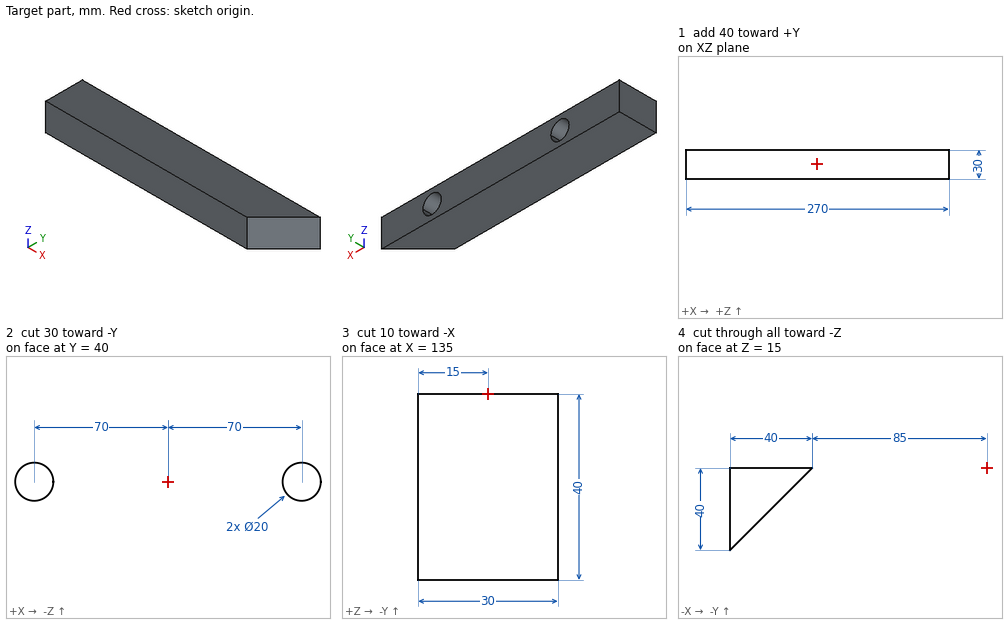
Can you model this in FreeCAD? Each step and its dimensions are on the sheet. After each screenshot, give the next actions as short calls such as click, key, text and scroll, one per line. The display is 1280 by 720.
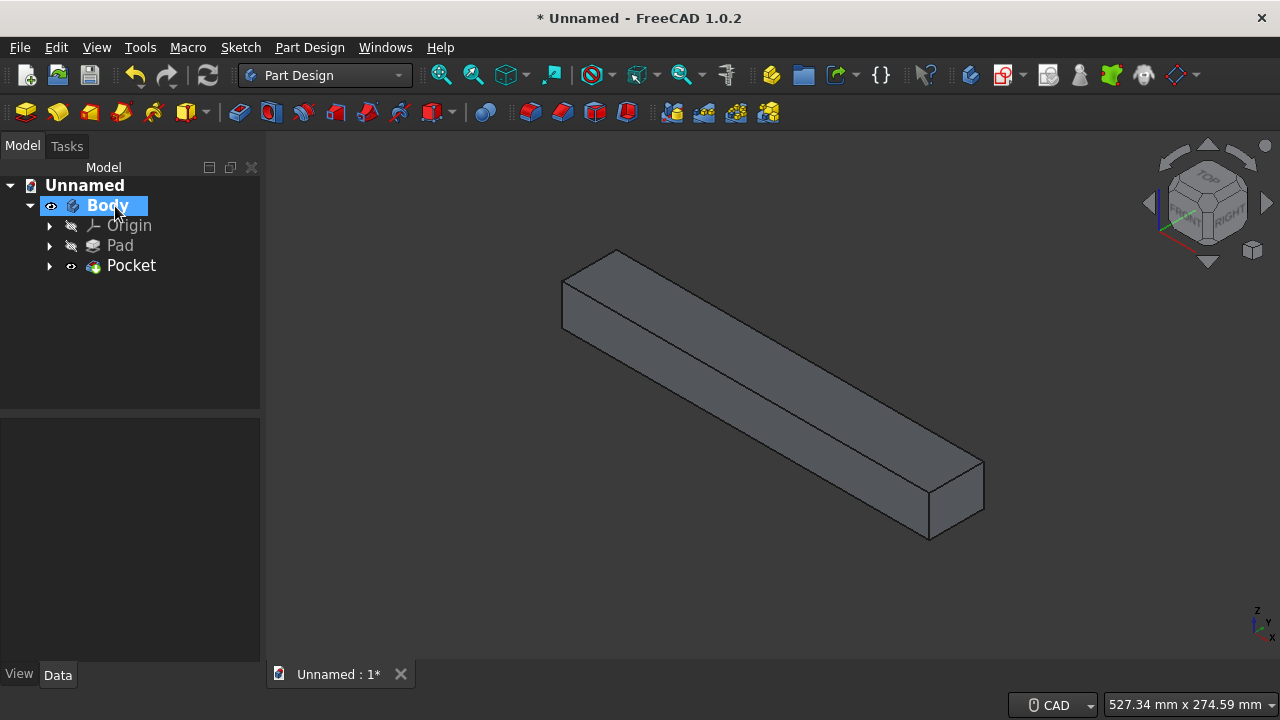
click(957, 500)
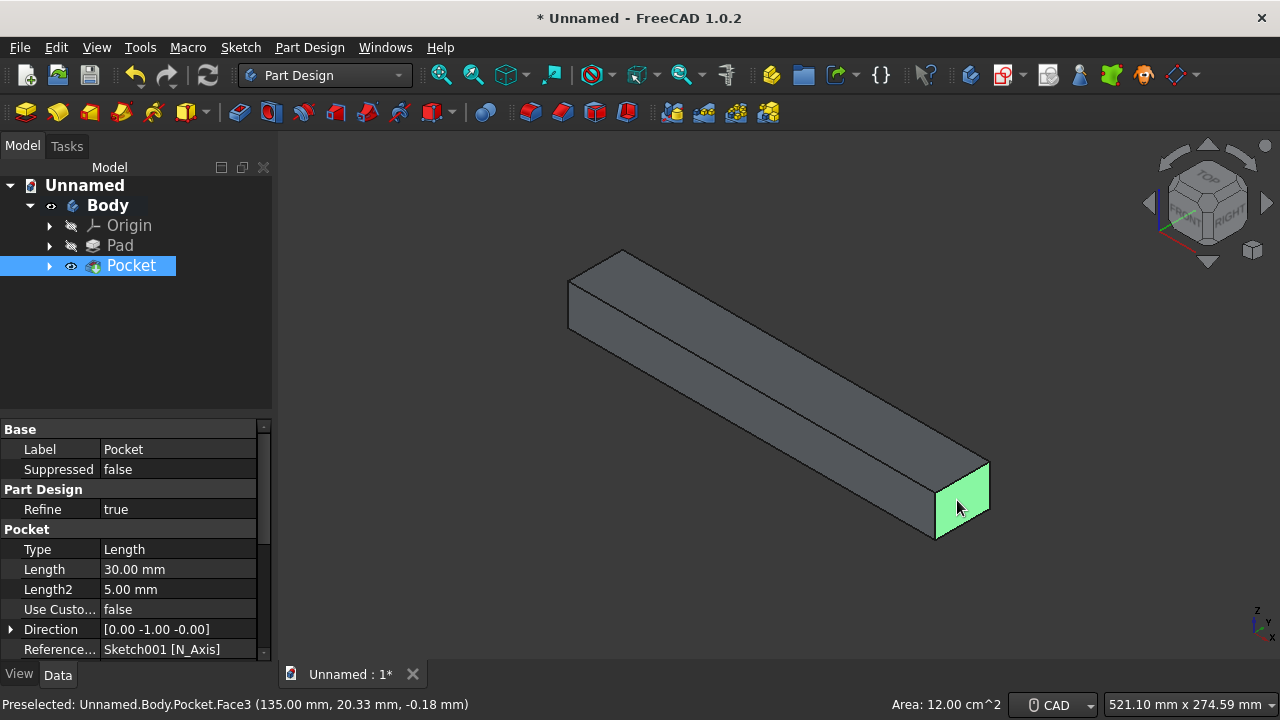
click(1004, 76)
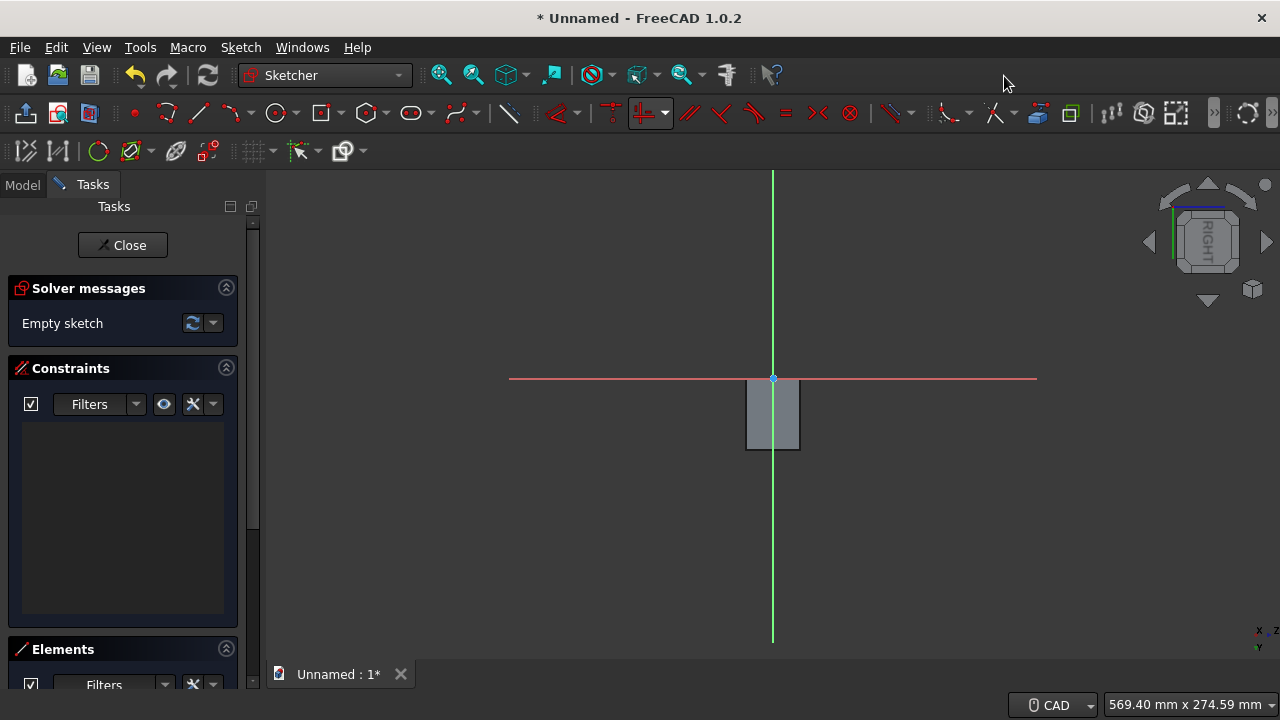
scroll(795, 415, up, 7)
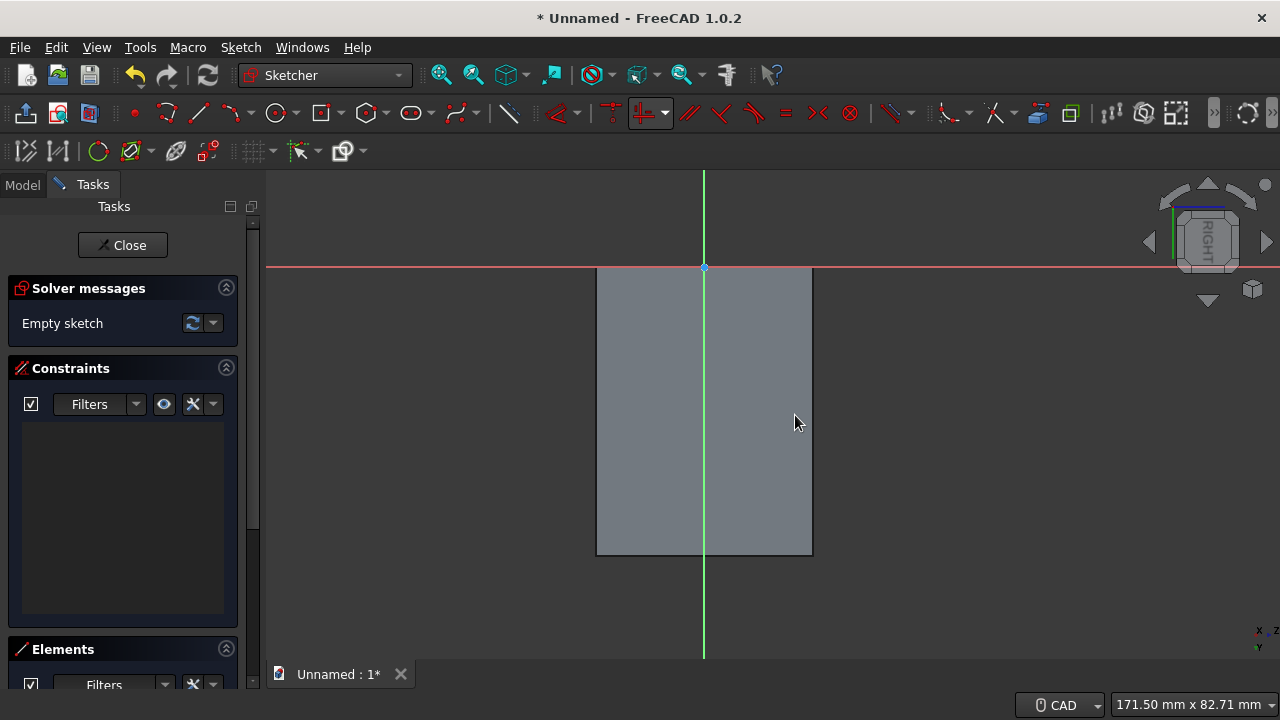
click(344, 114)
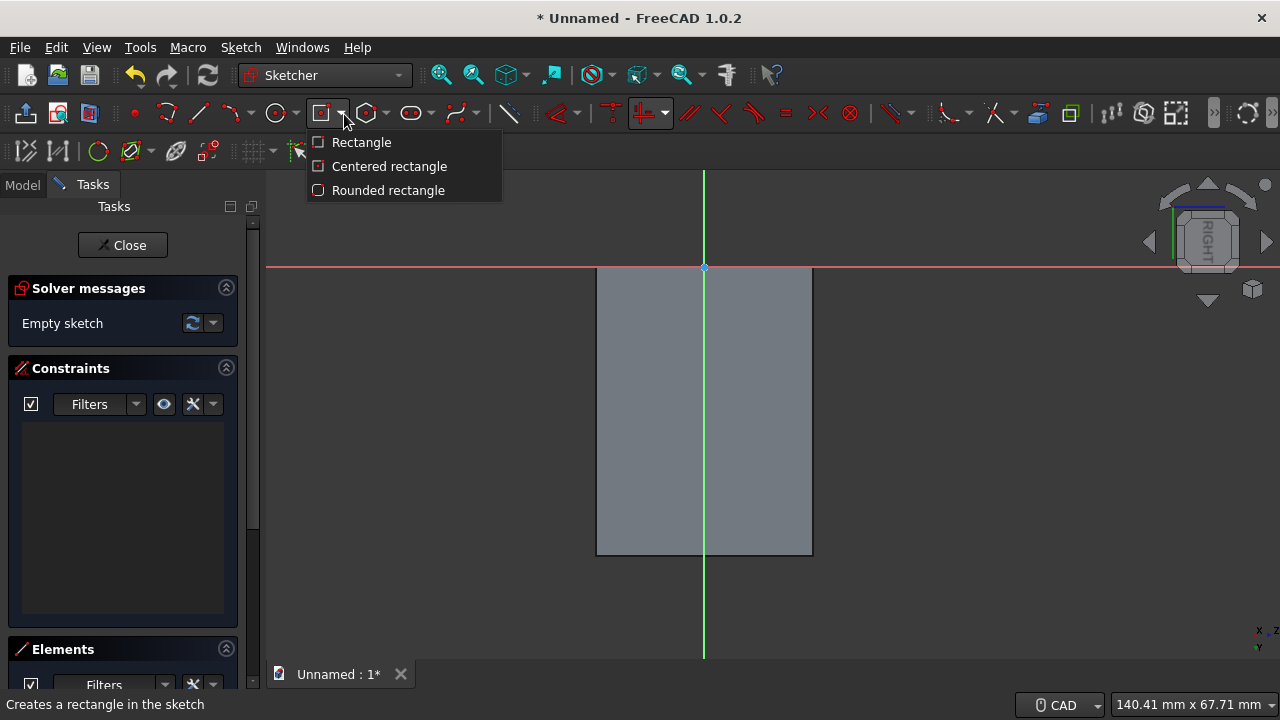
click(404, 142)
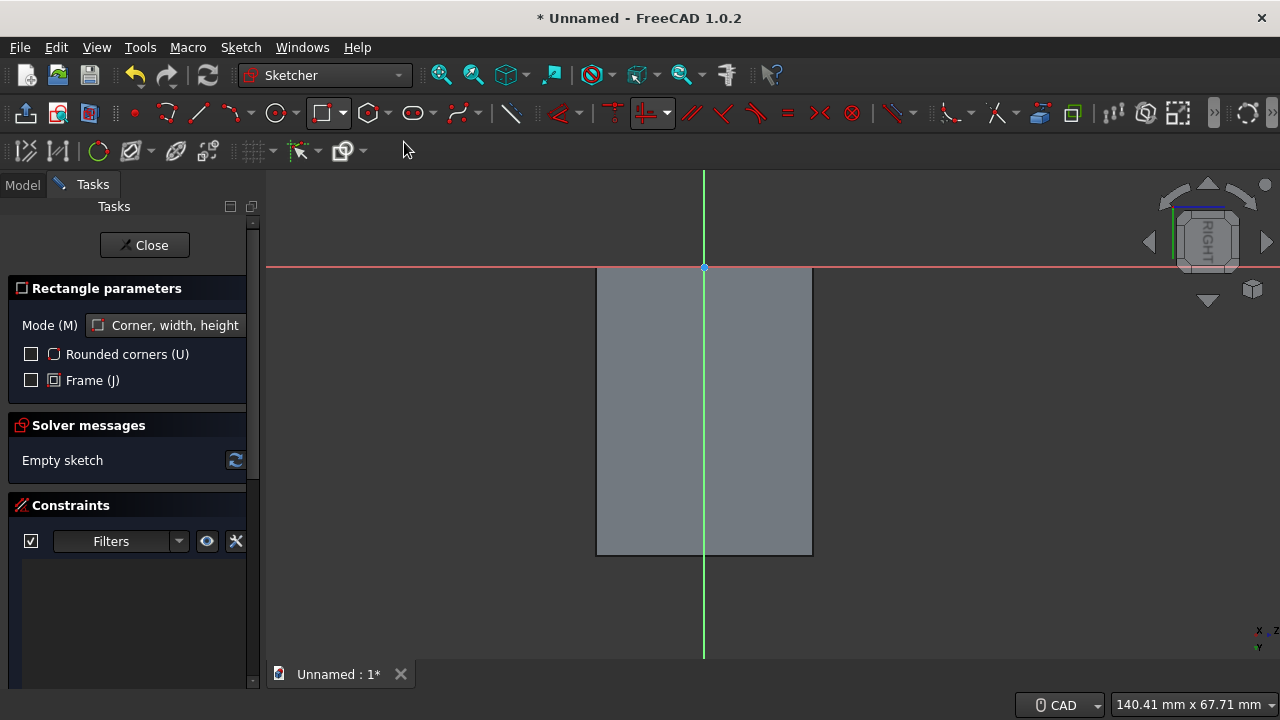
click(596, 267)
move(813, 556)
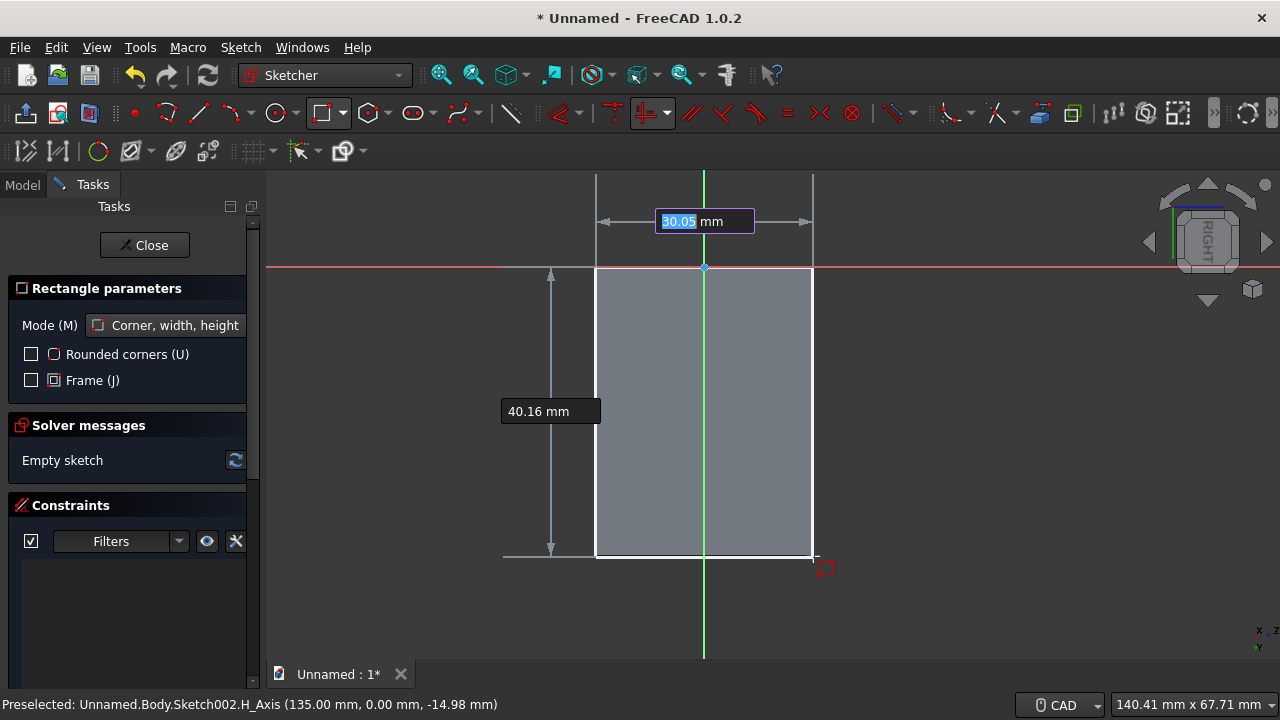
text(30)
key(Tab)
text(40)
key(Return)
key(Escape)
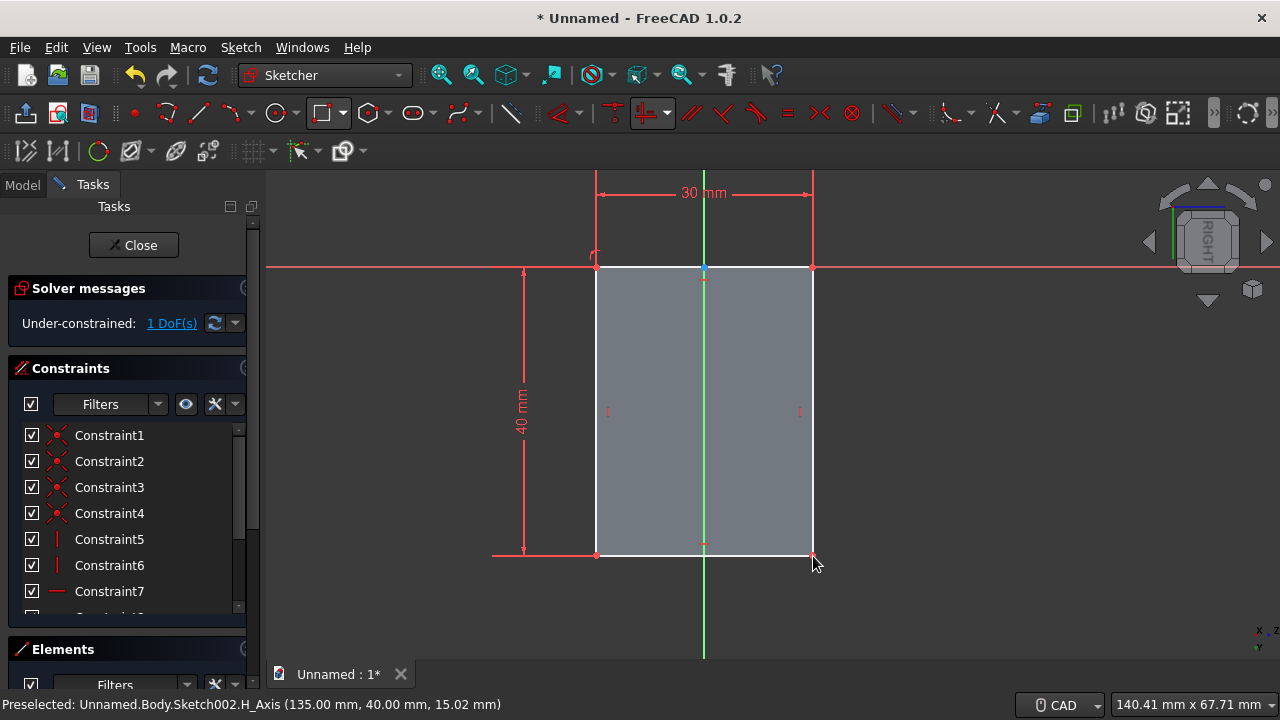
click(558, 114)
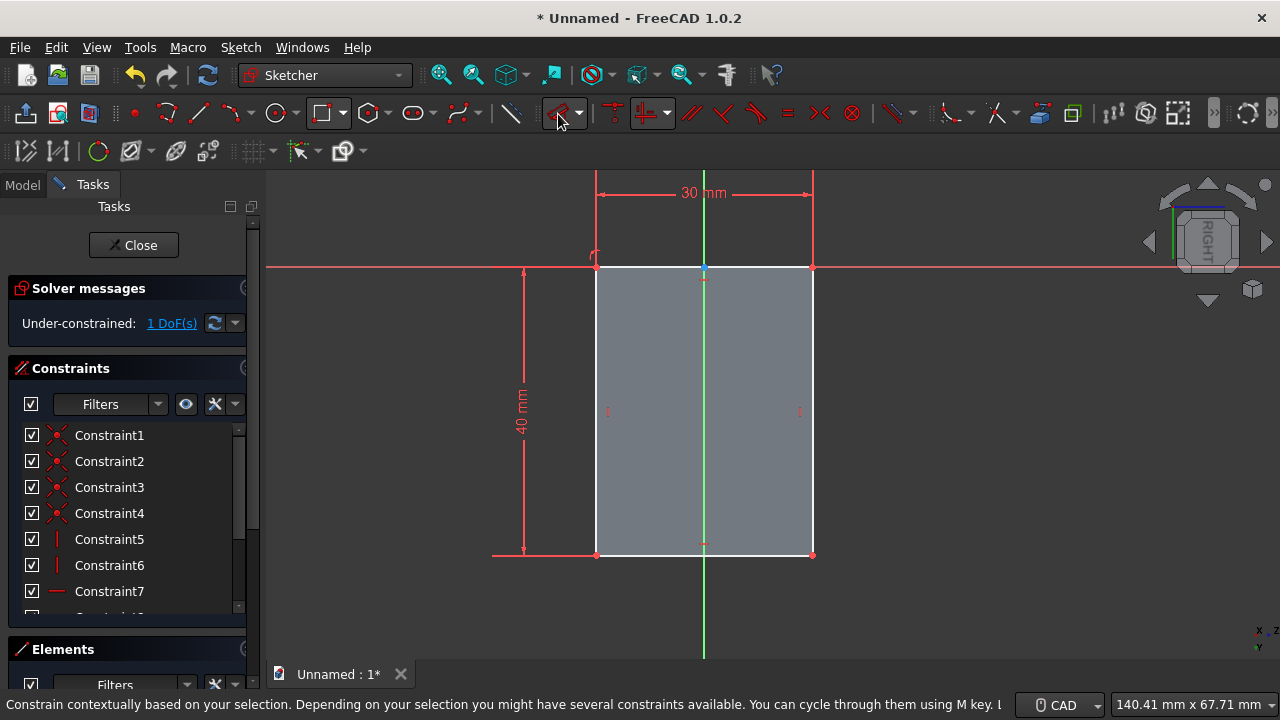
click(596, 267)
click(650, 233)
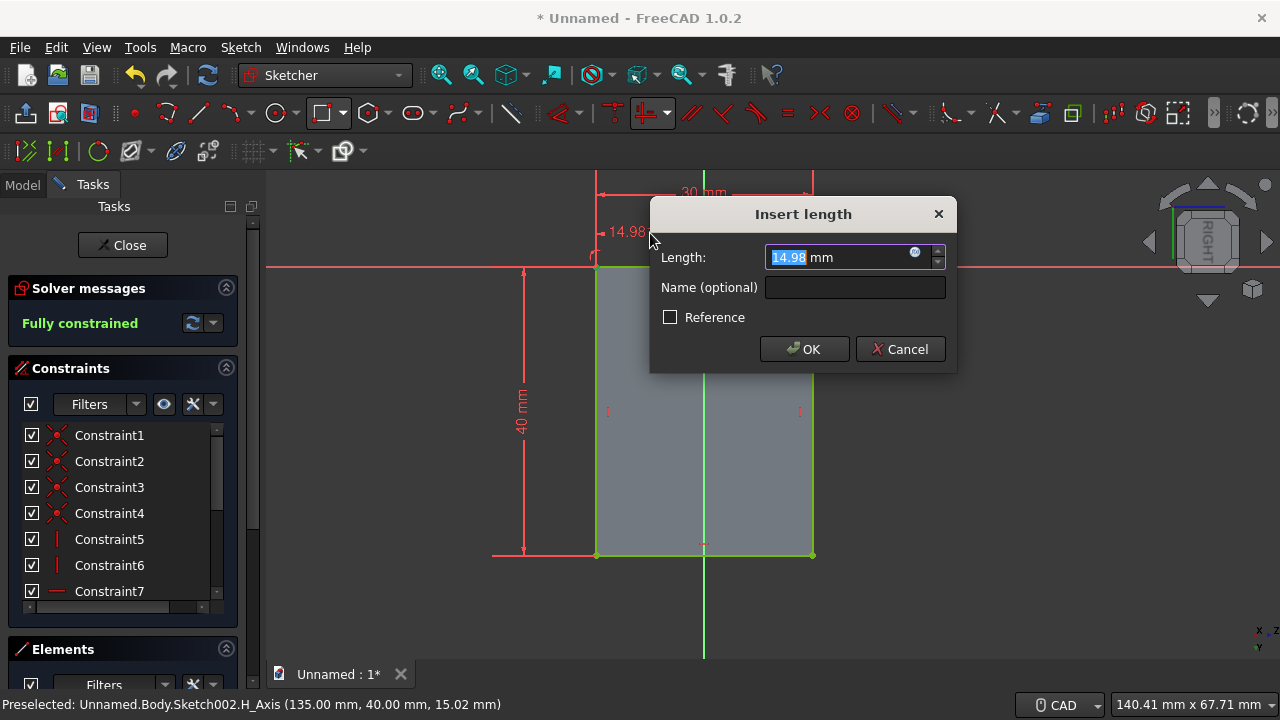
text(15)
key(Return)
key(Escape)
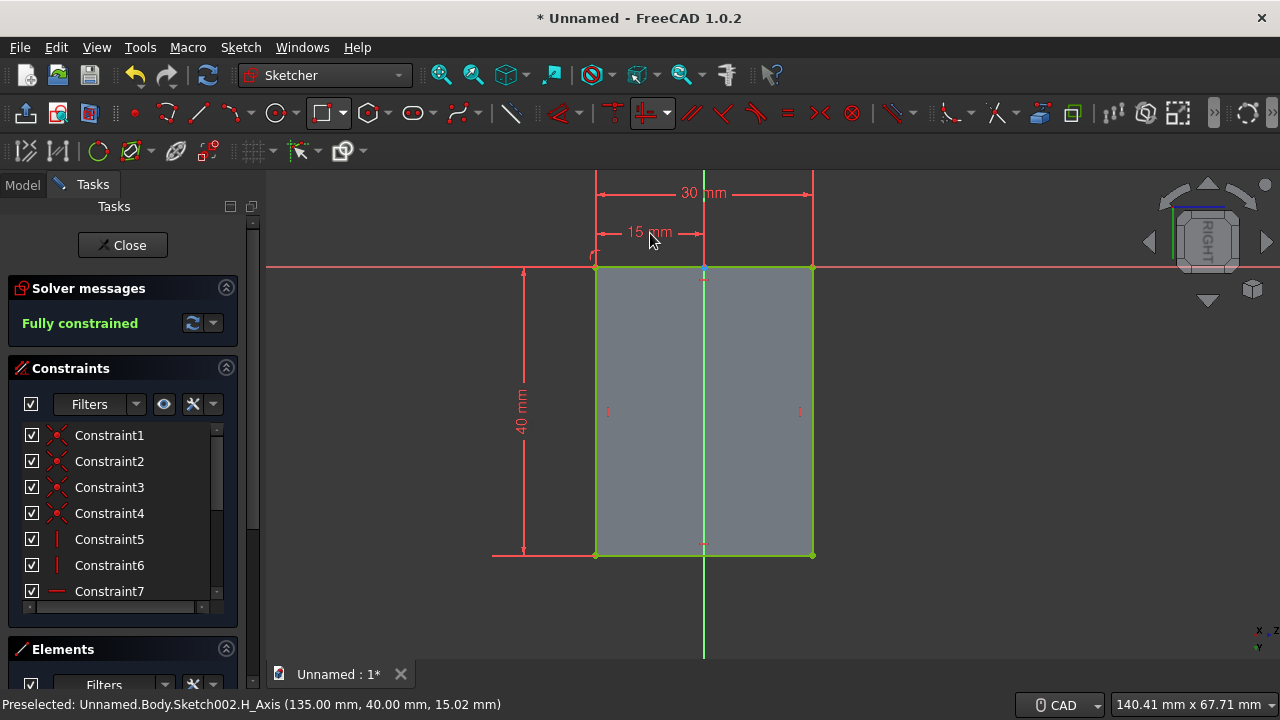
click(123, 245)